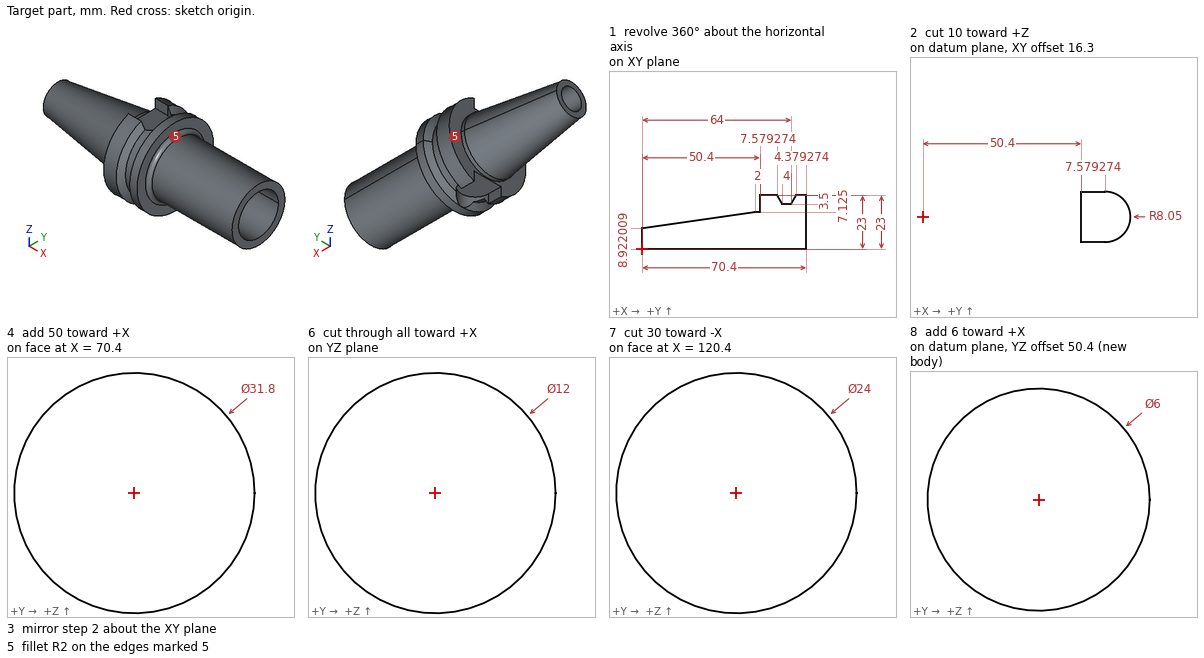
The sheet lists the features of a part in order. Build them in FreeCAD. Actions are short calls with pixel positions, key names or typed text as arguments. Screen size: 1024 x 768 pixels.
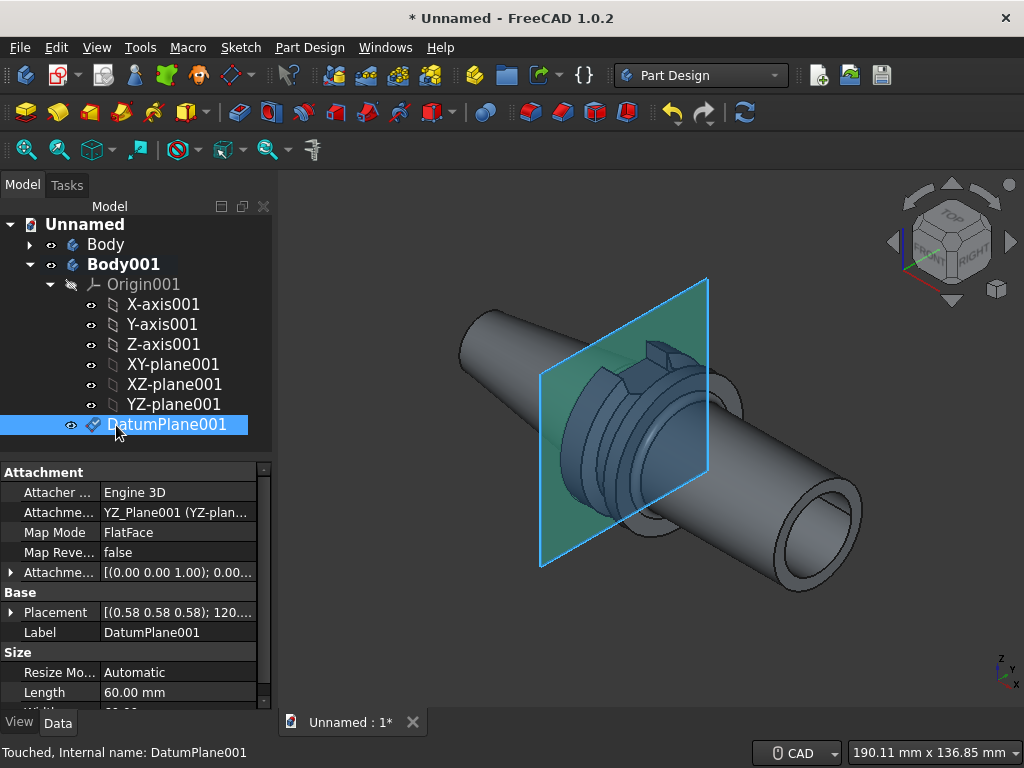
click(58, 76)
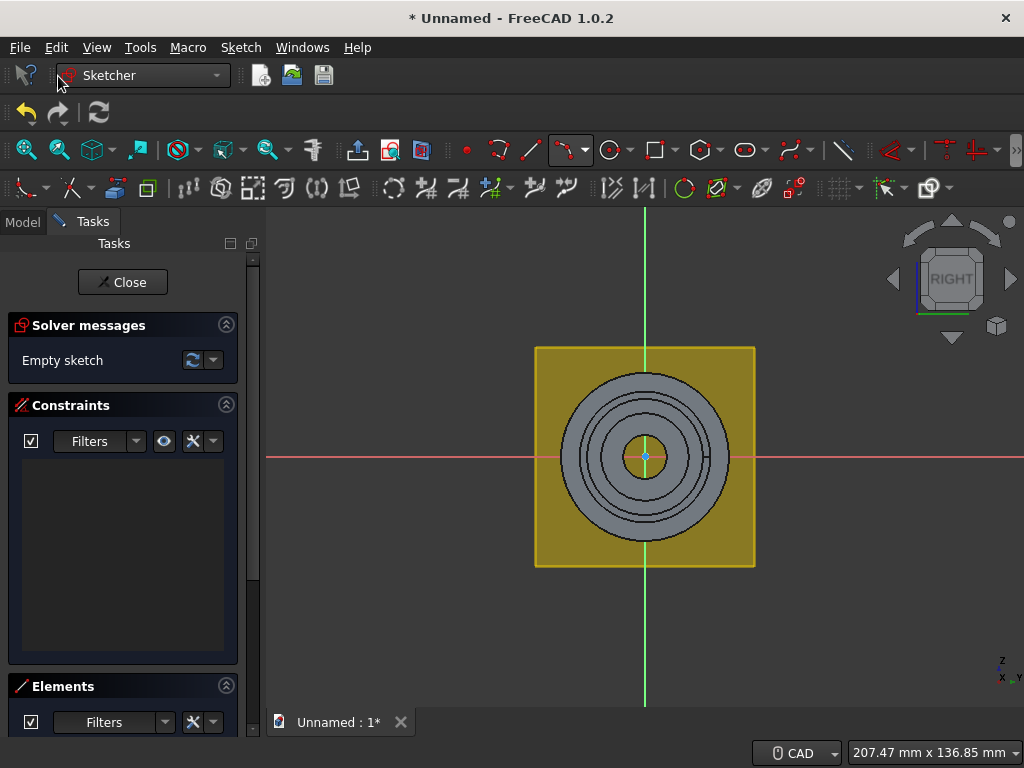
scroll(650, 457, up, 13)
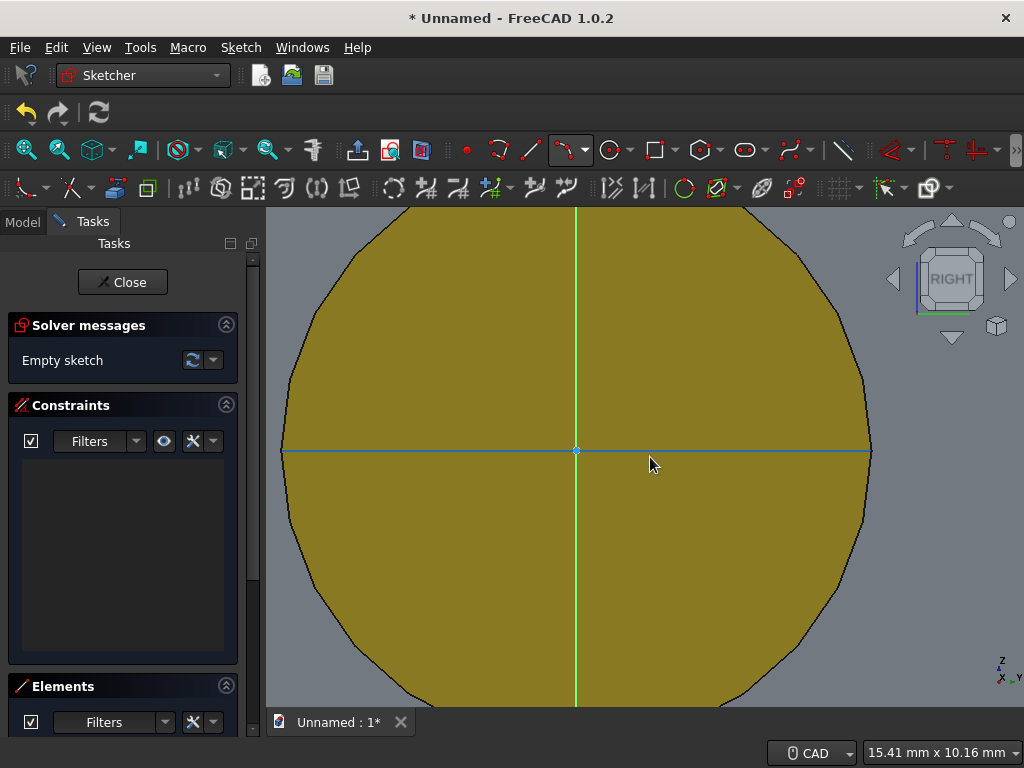
click(610, 150)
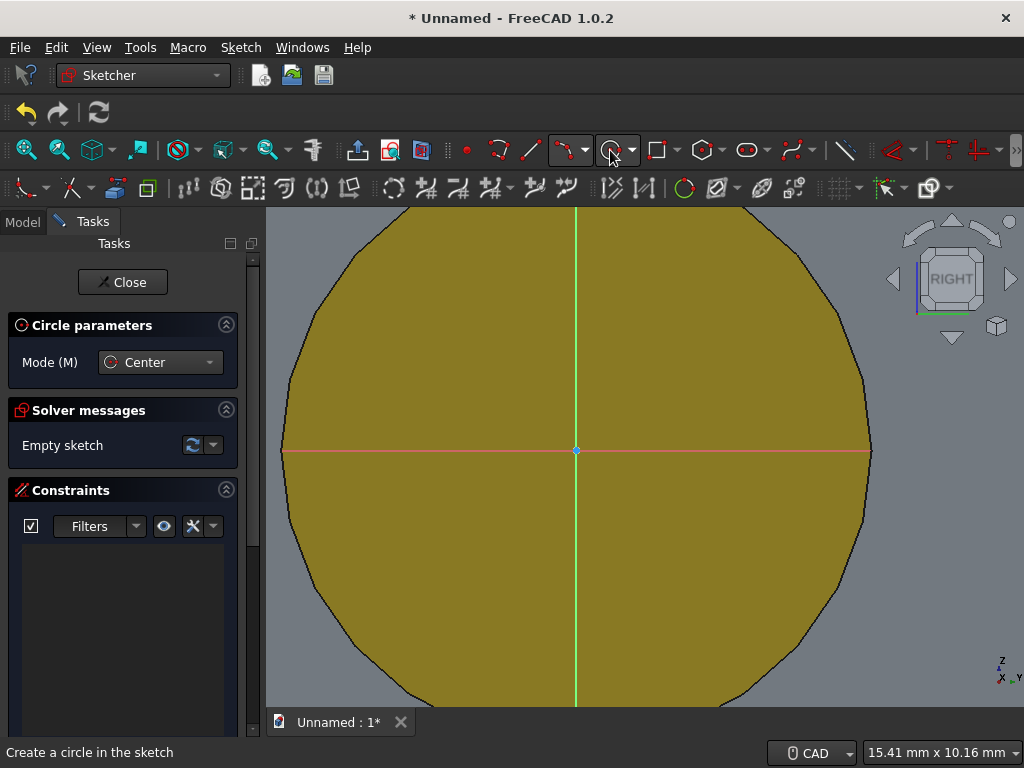
click(576, 451)
move(681, 346)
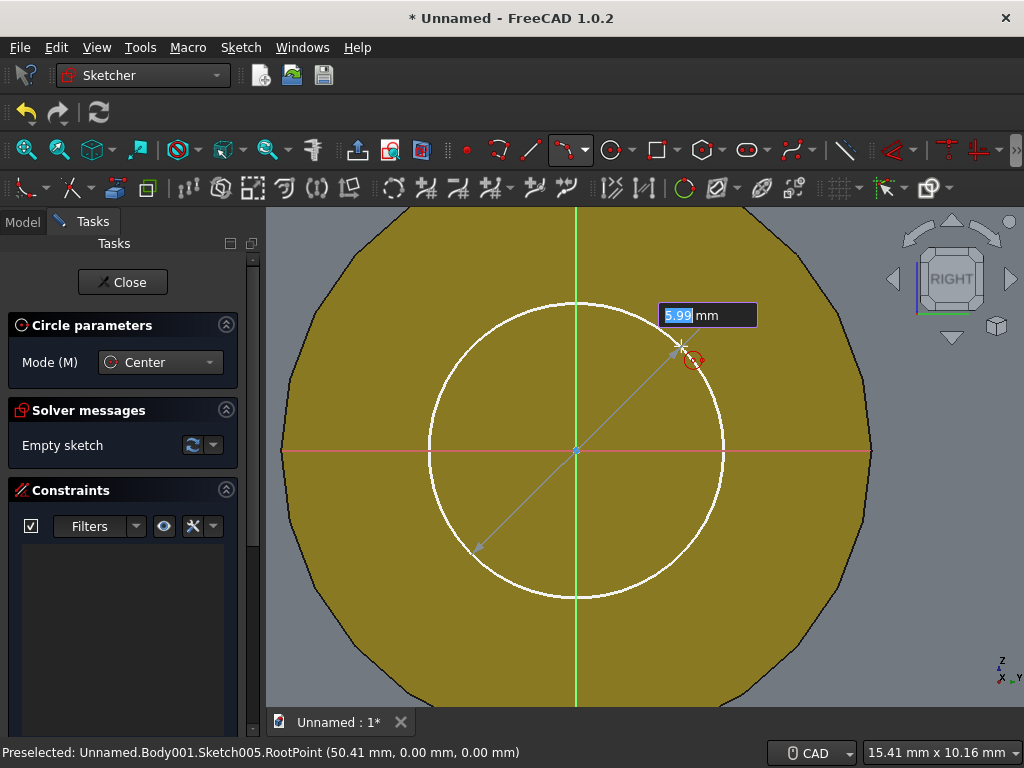
text(6)
key(Return)
key(Escape)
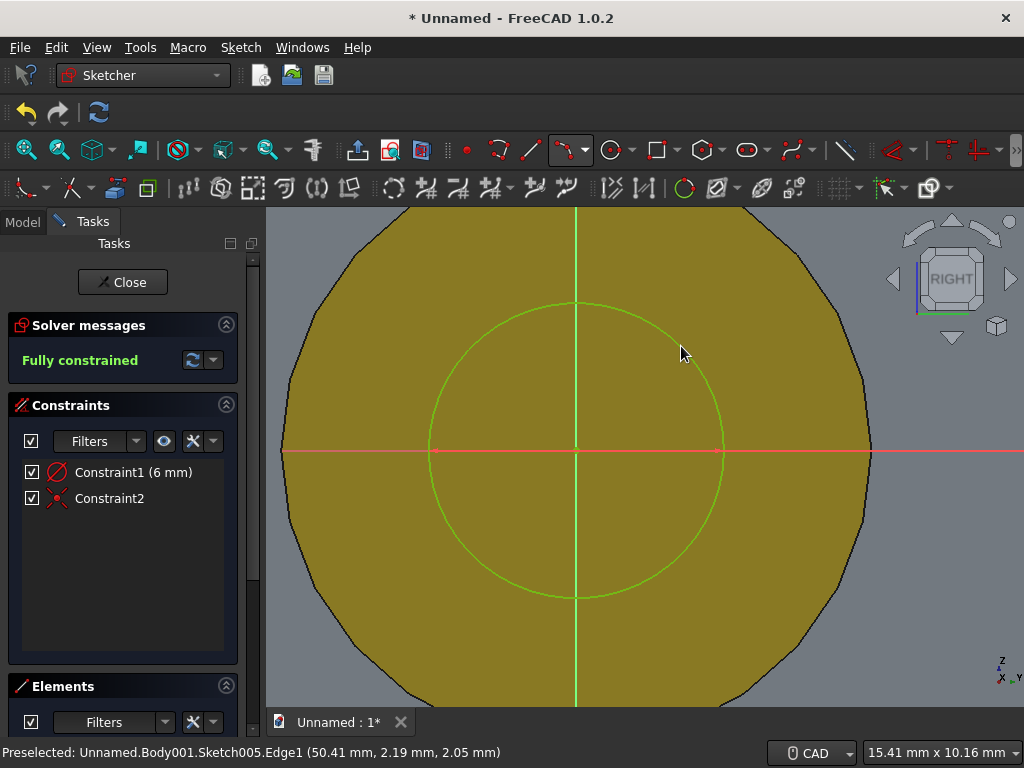
click(123, 282)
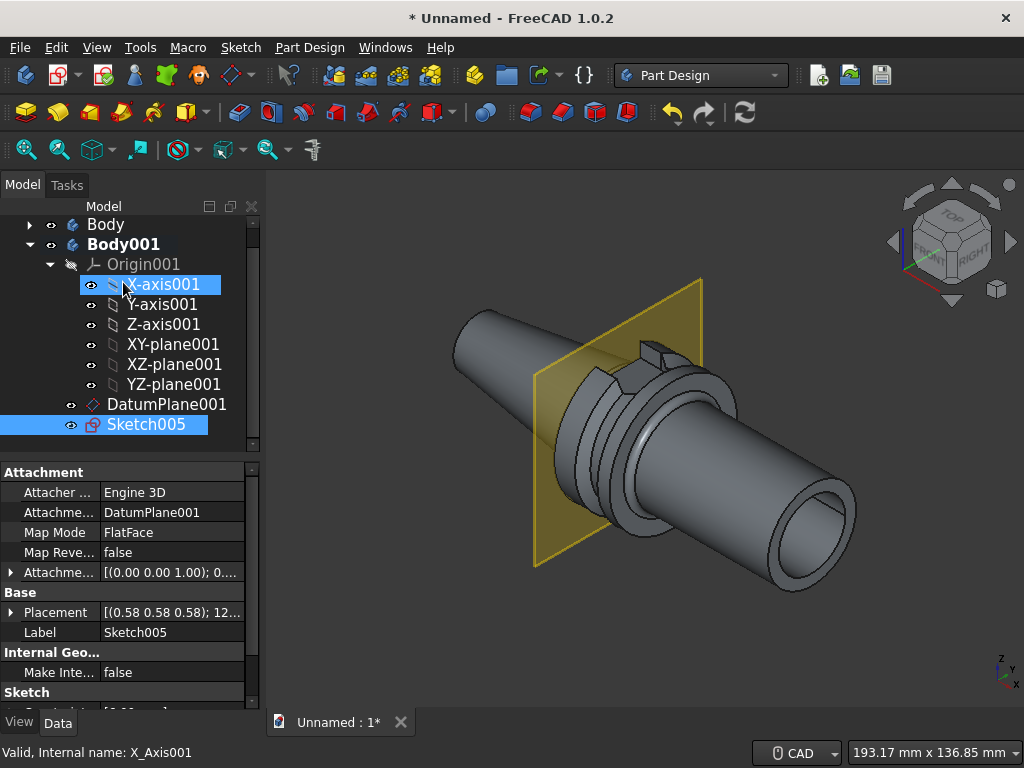
click(26, 112)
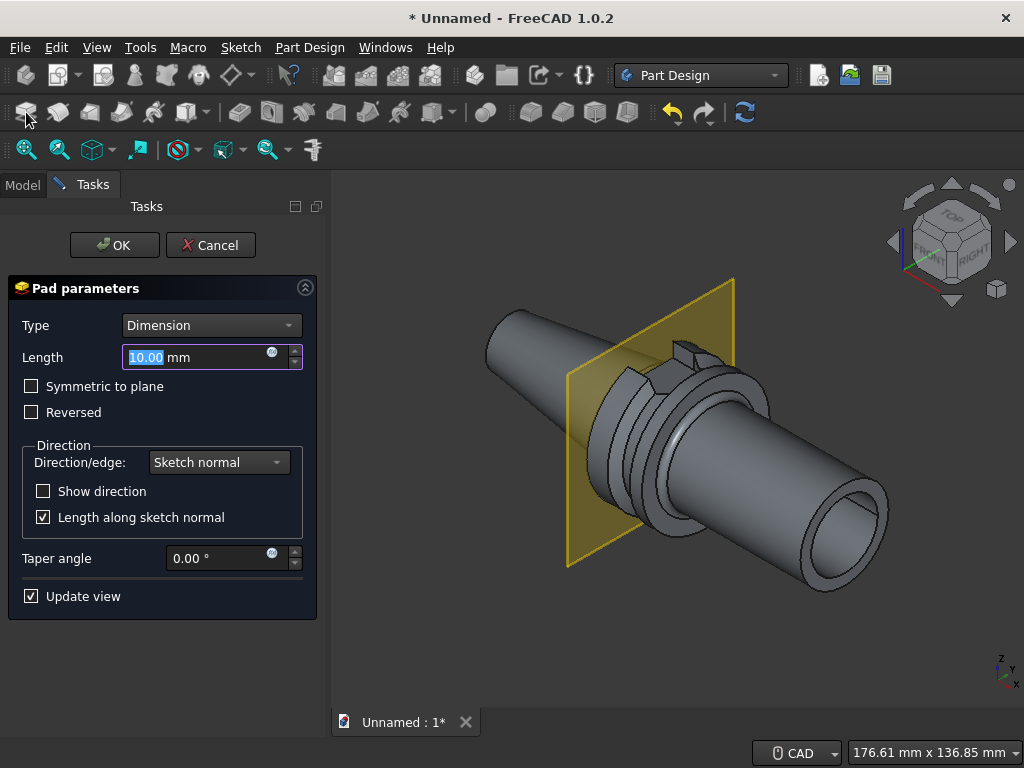
text(6)
key(Tab)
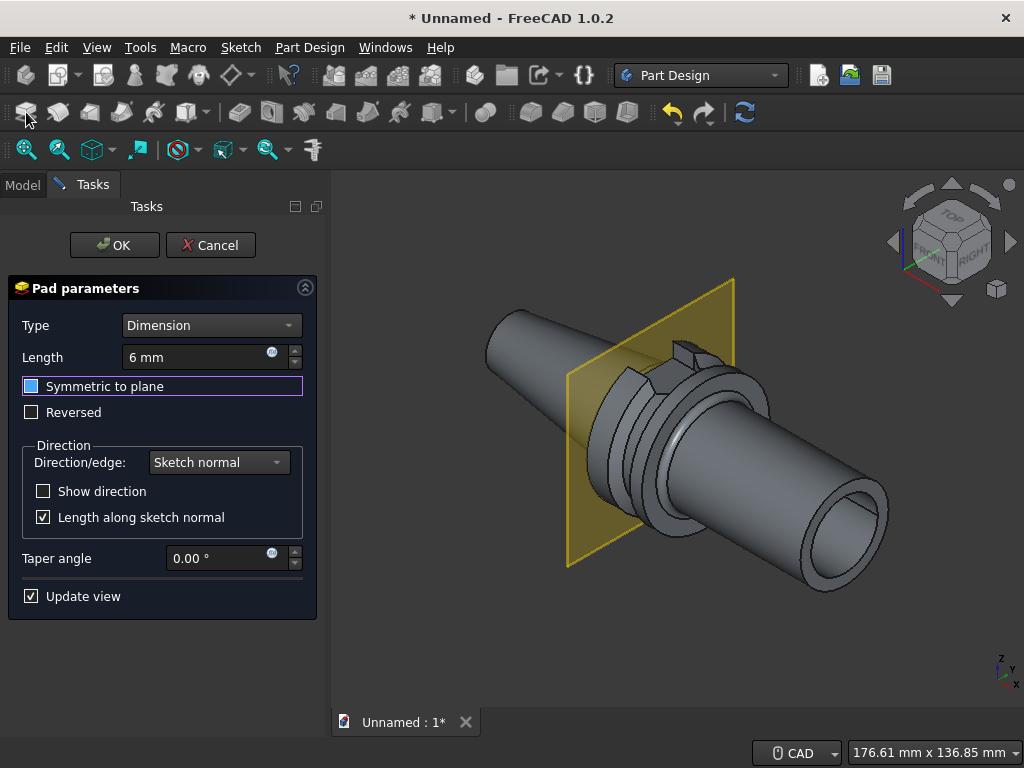
click(115, 245)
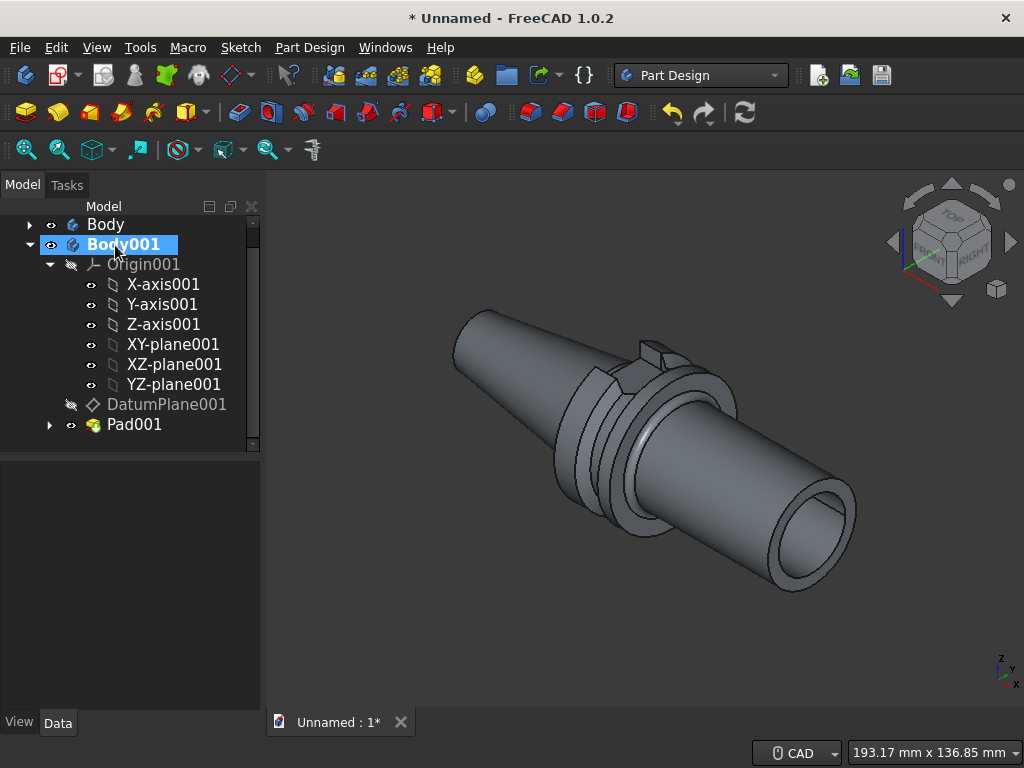
key(v)
key(f)